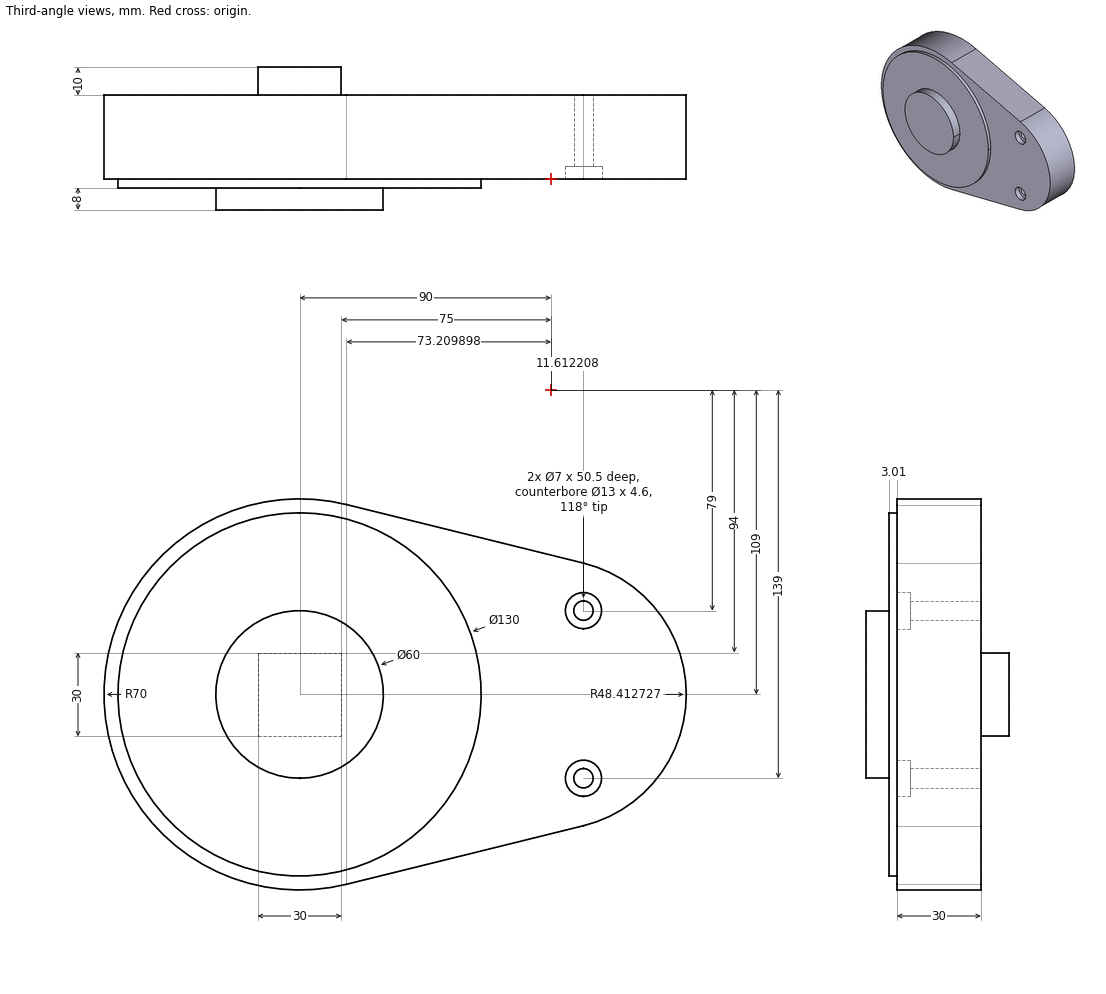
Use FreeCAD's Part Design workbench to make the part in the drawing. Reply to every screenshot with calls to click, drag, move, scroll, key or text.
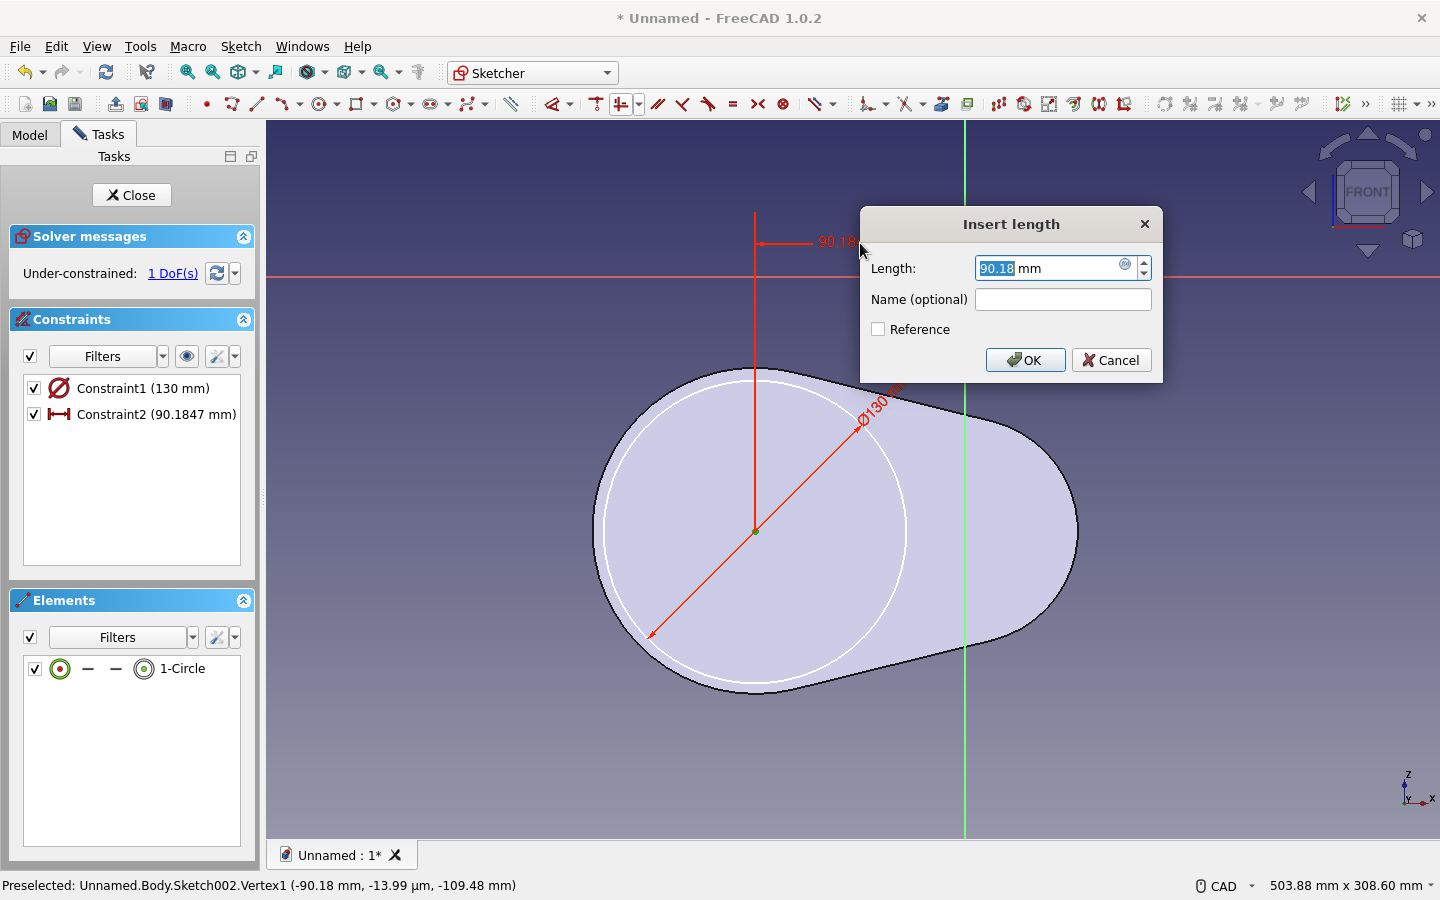
text(90)
key(Return)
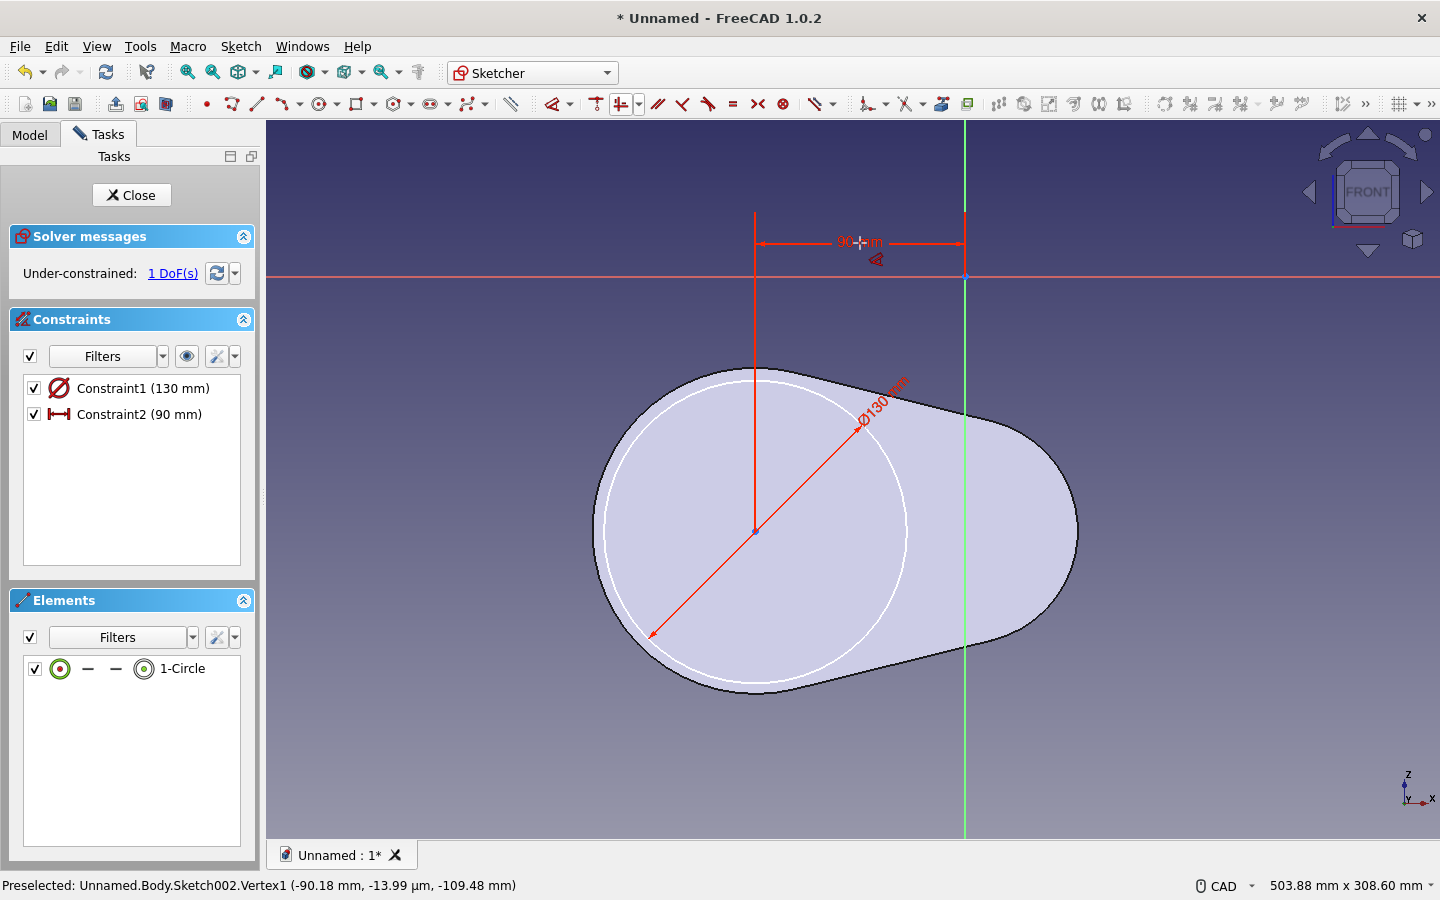
click(755, 532)
click(999, 404)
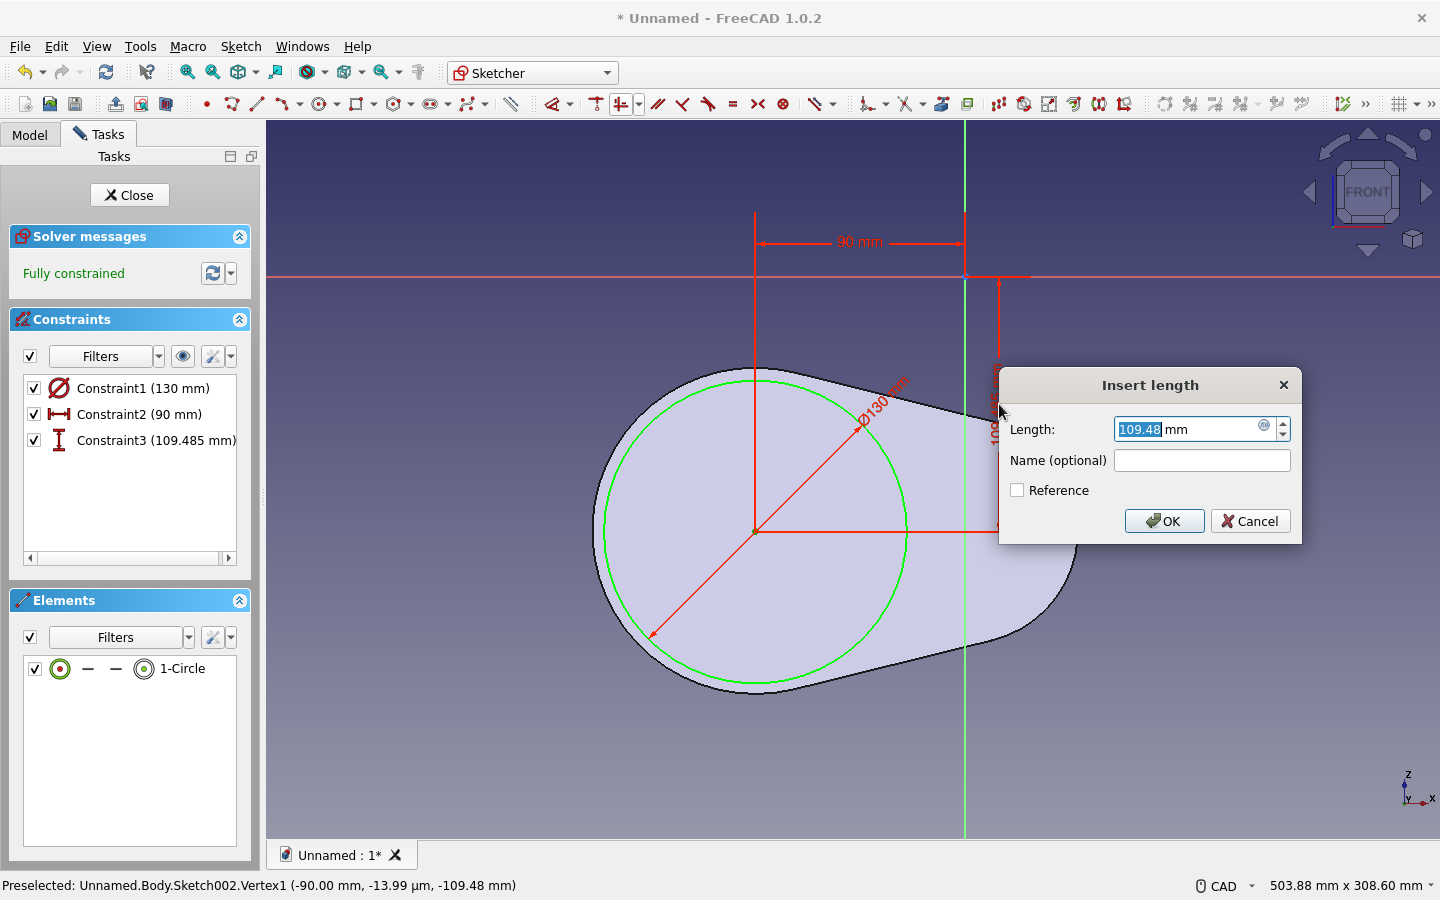
text(109)
key(Return)
key(Escape)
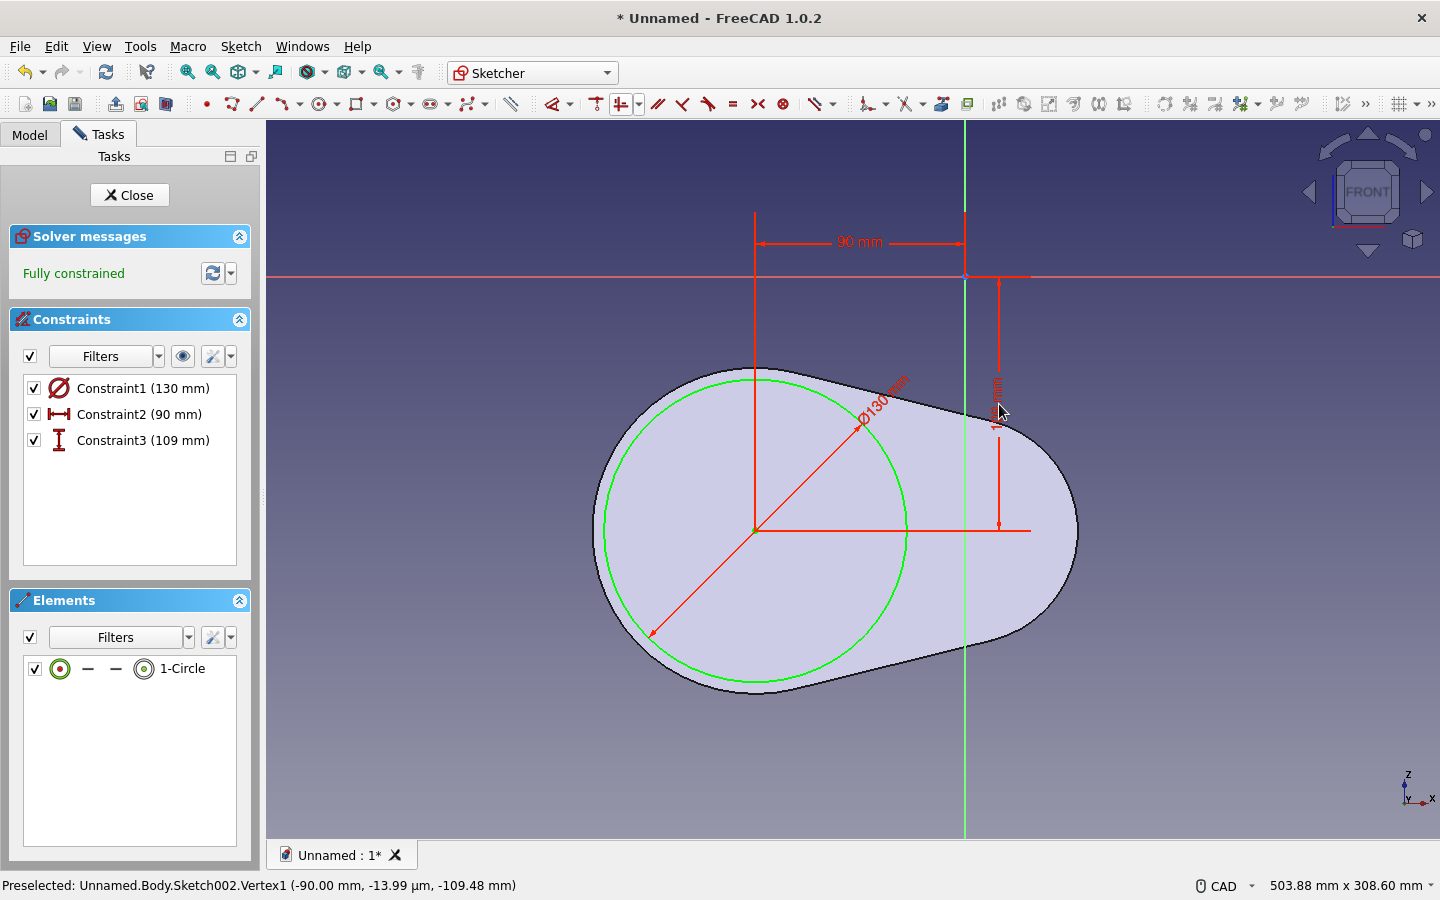
click(130, 195)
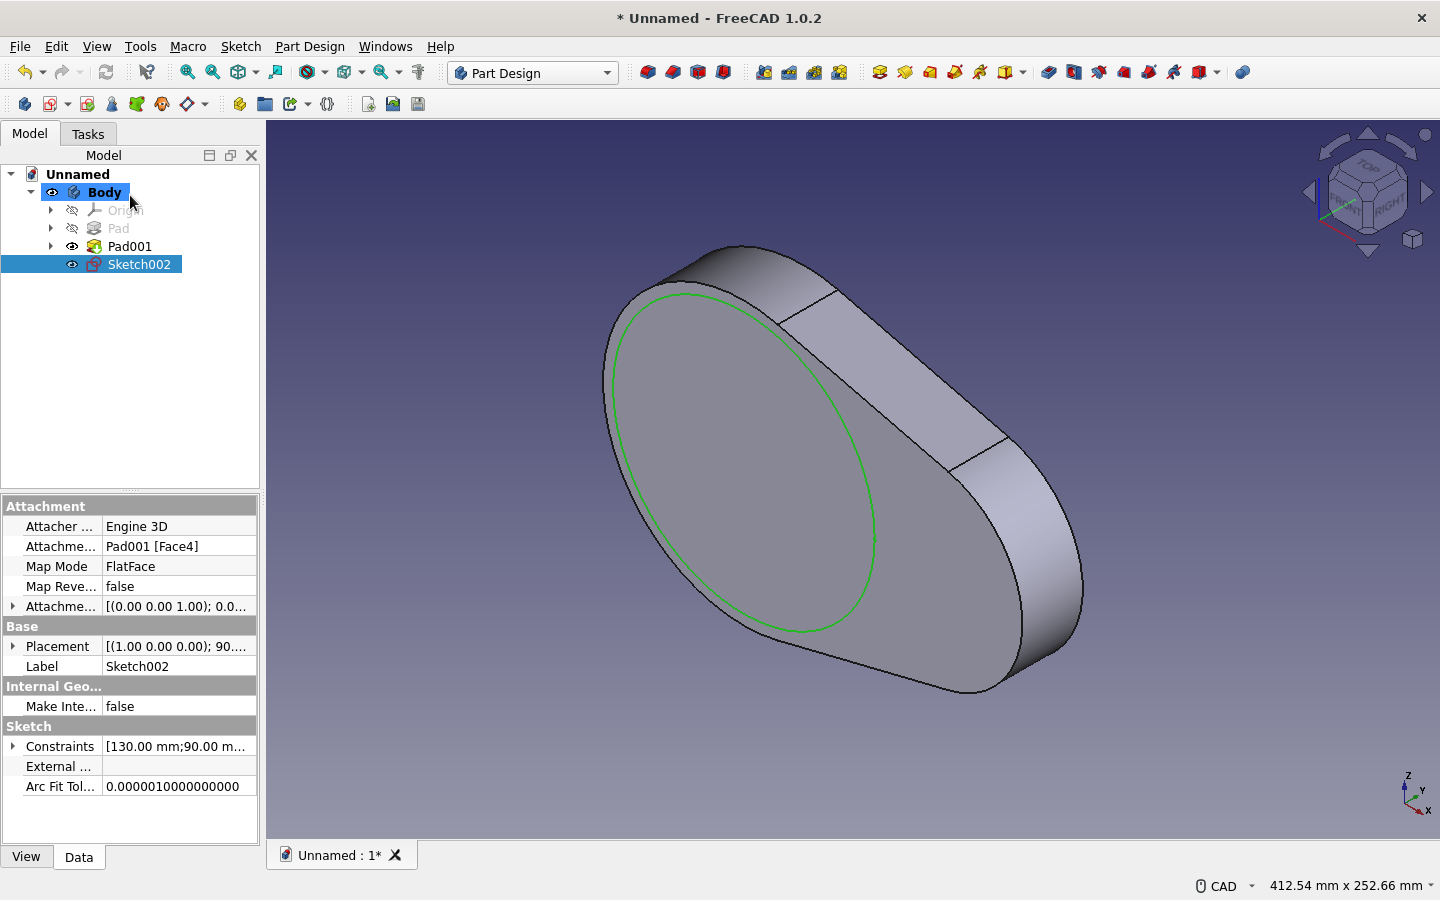
click(880, 72)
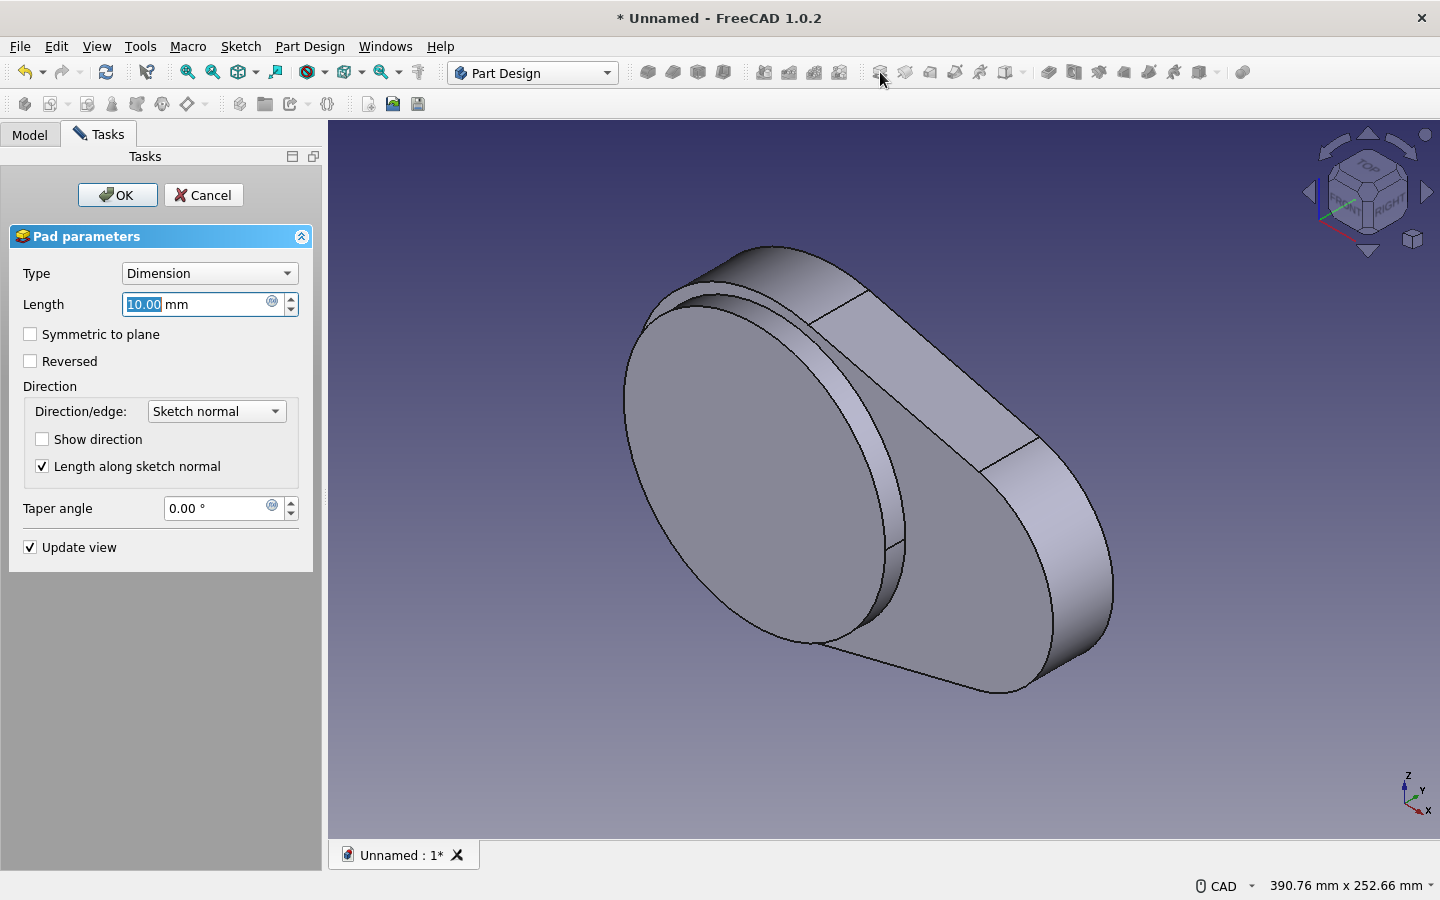
text(3.01)
key(Tab)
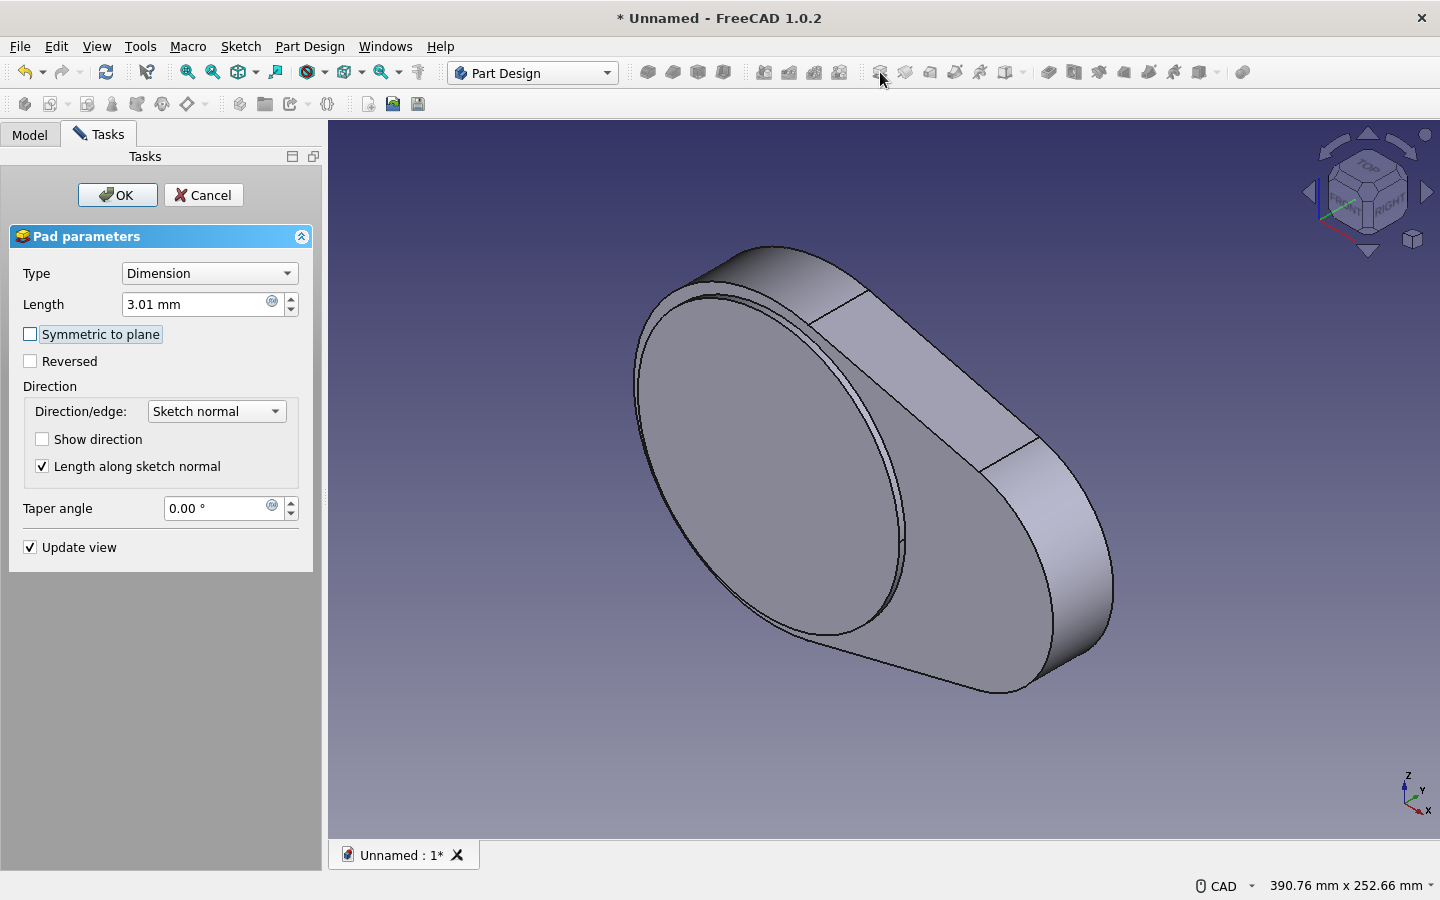
click(118, 195)